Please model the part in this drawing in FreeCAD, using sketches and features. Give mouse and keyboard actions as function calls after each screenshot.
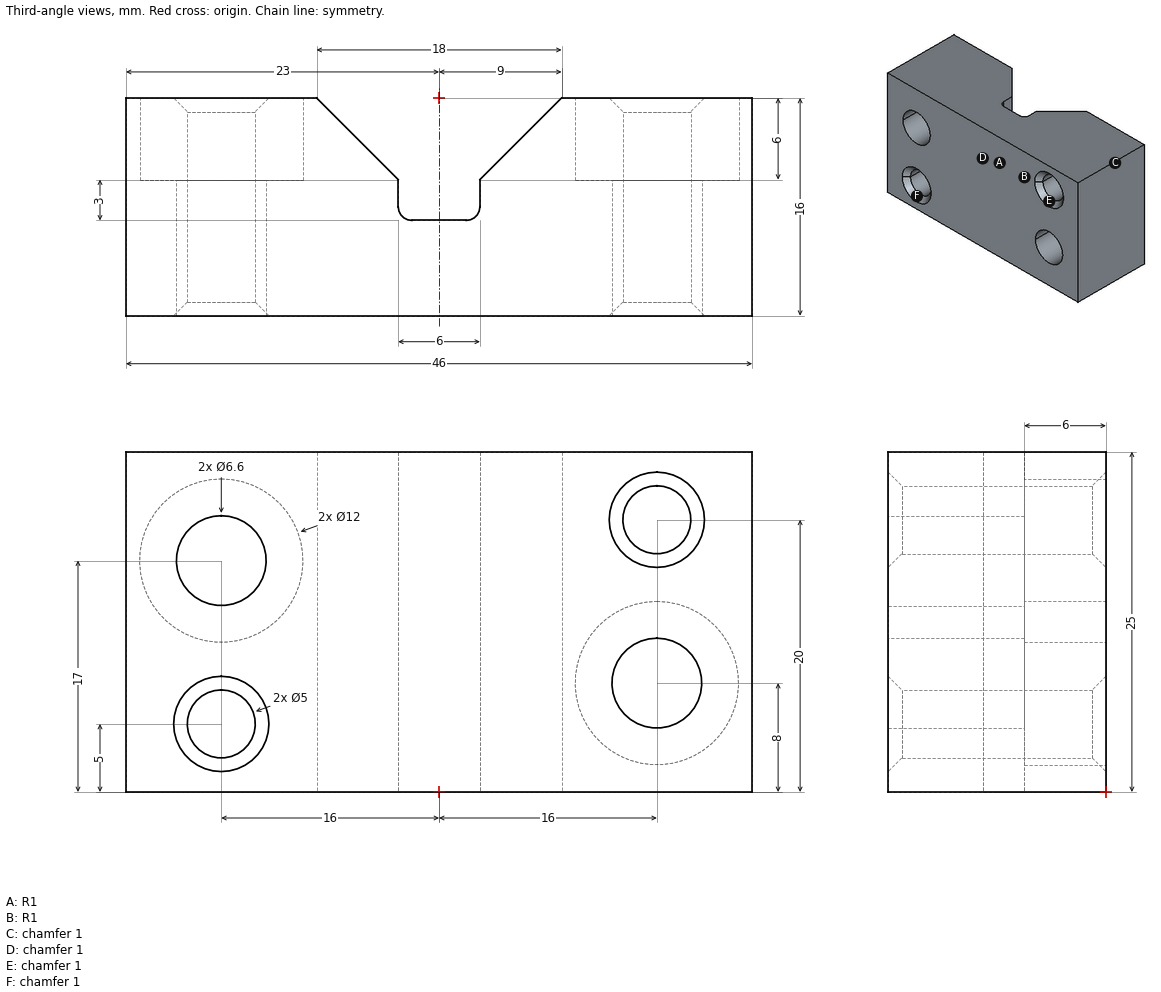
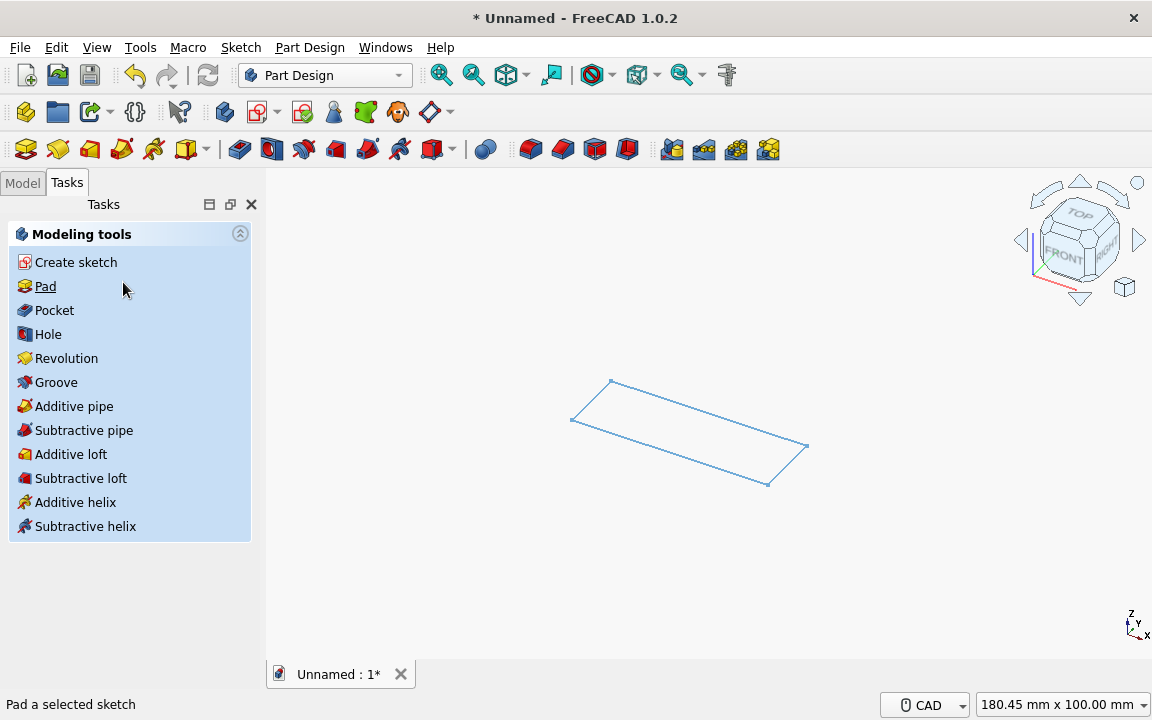
click(26, 150)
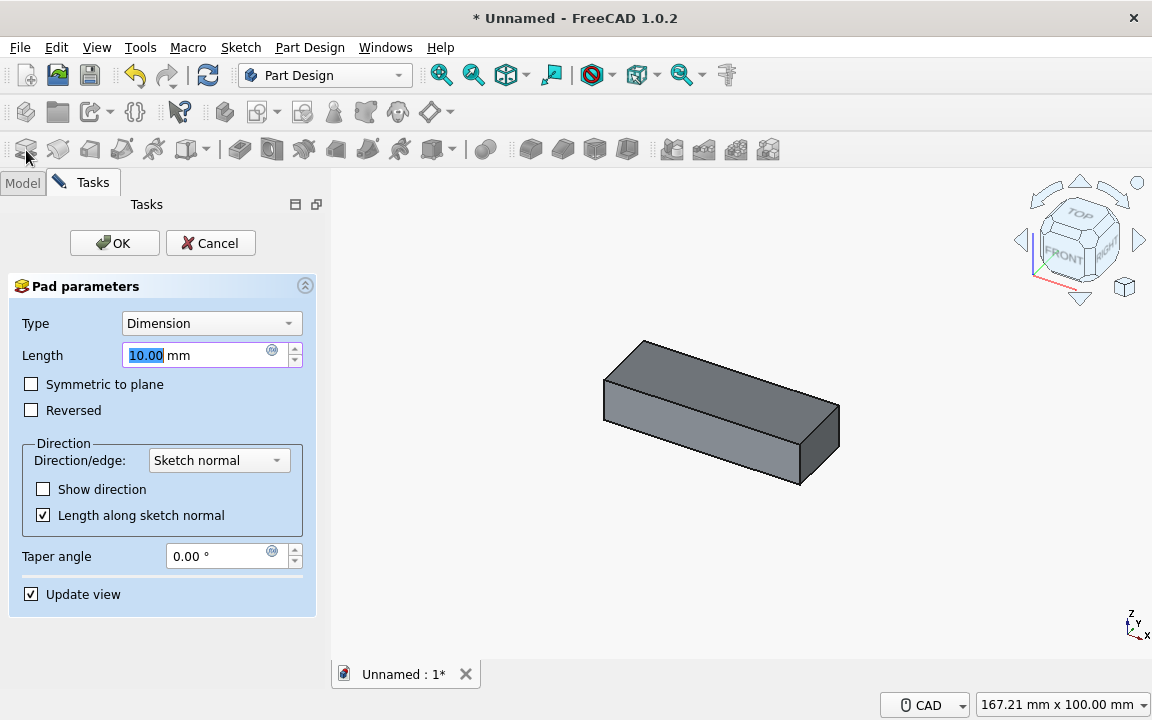
text(25)
key(Tab)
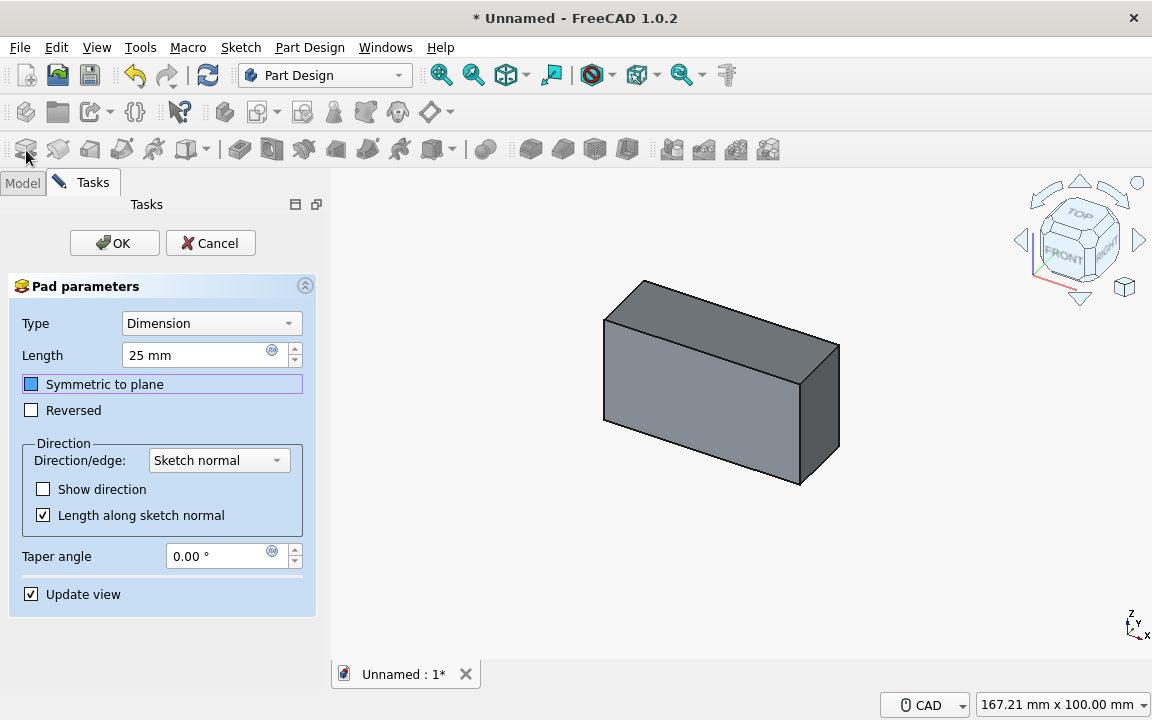
click(115, 243)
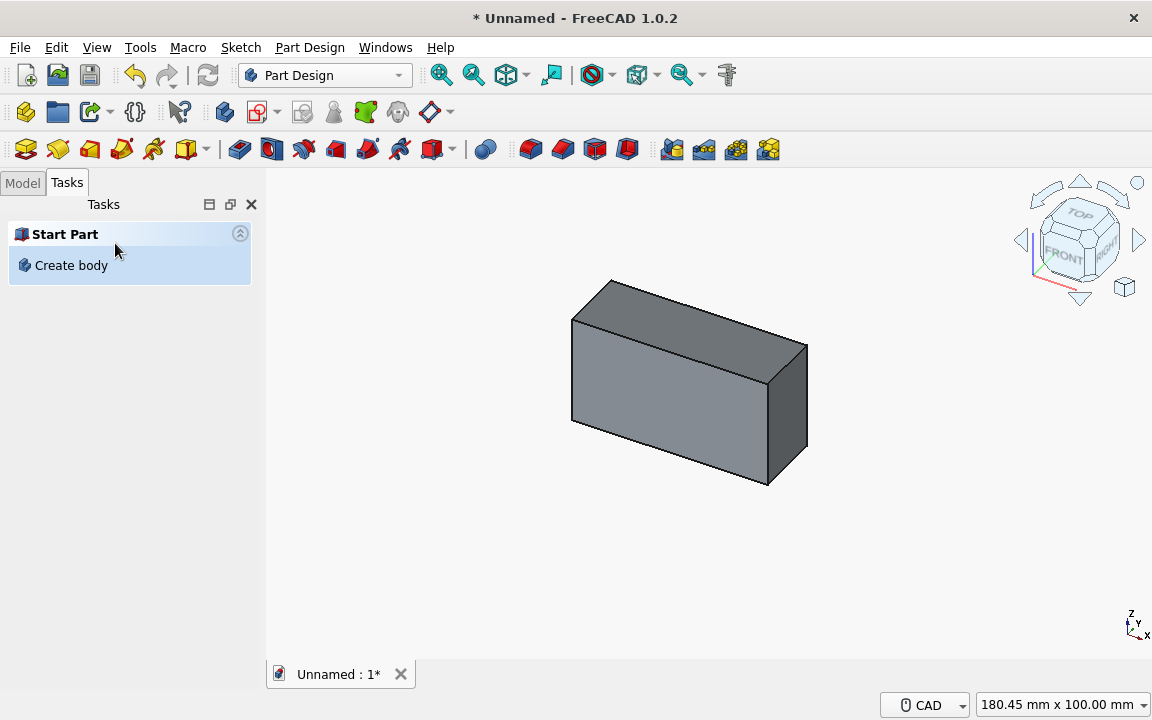
click(442, 76)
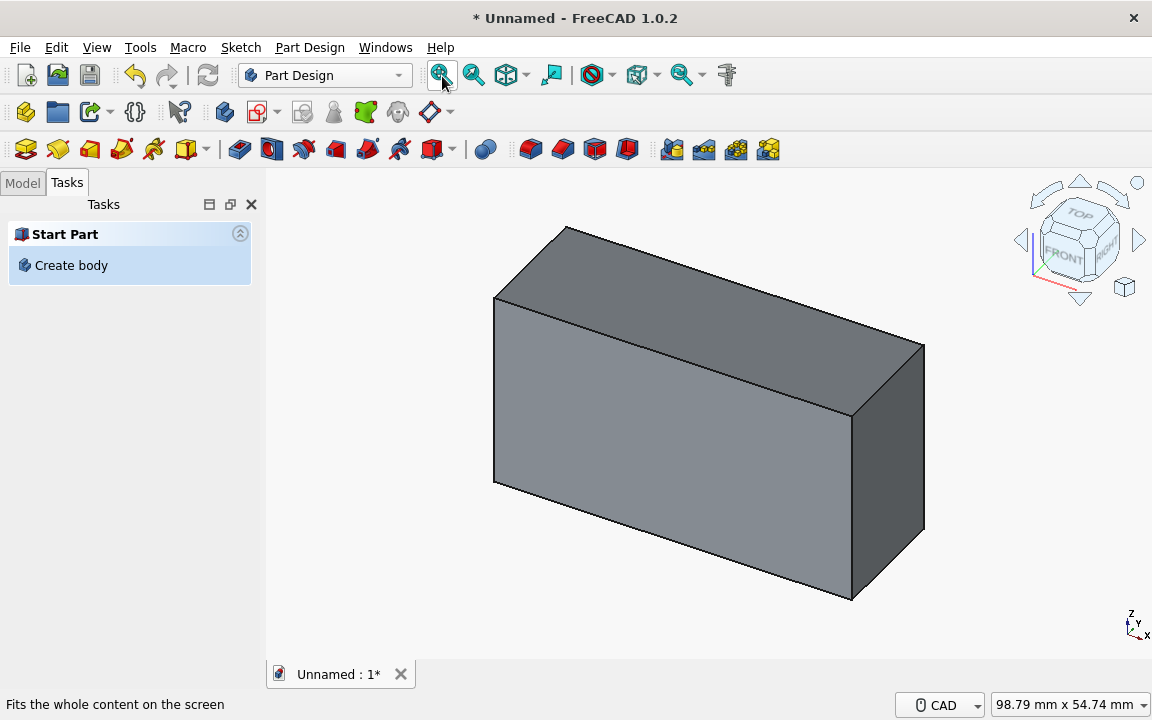
click(811, 354)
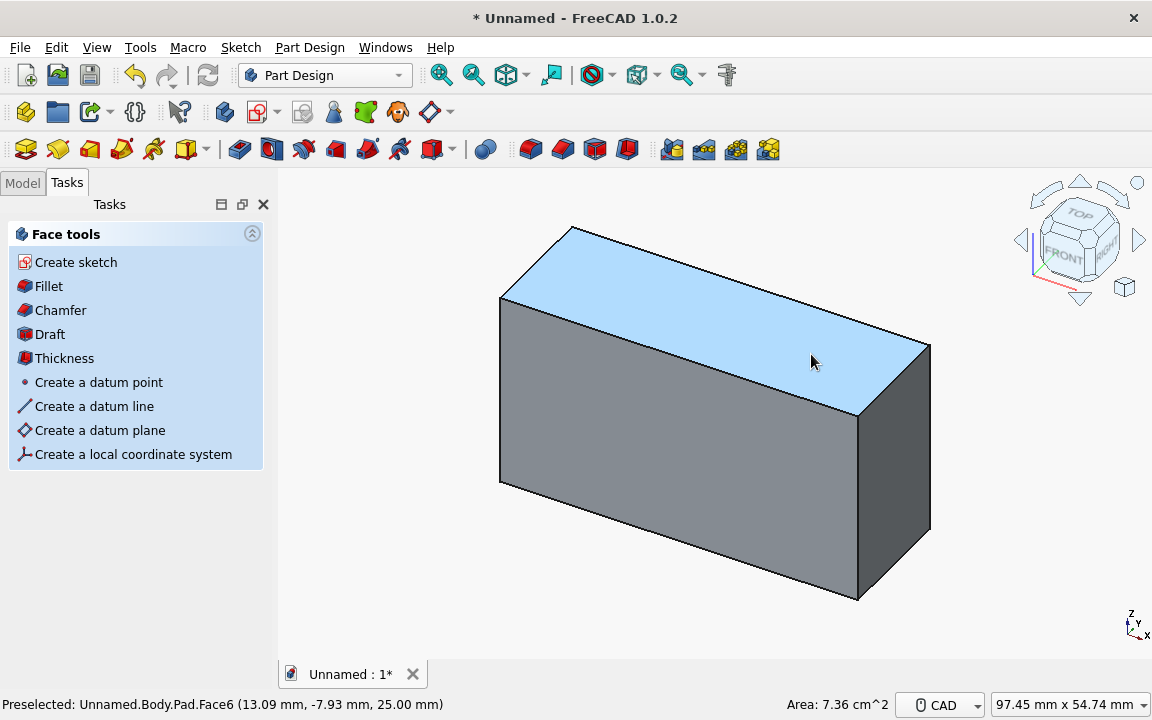
click(258, 112)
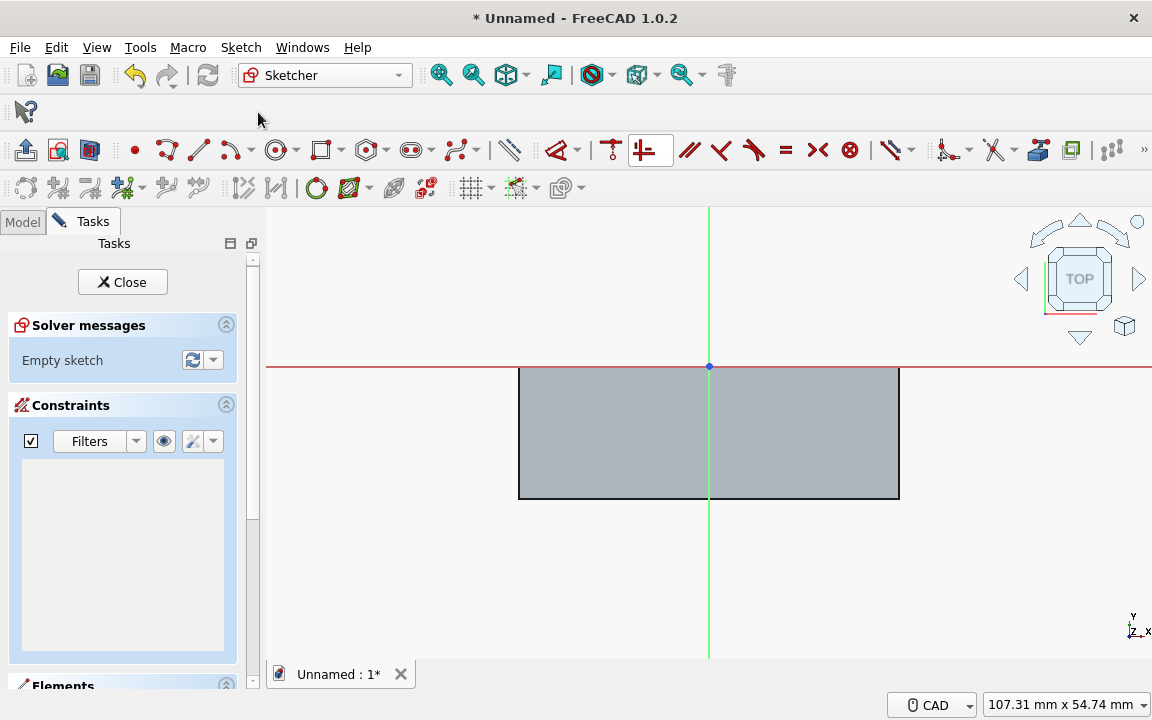
scroll(739, 392, up, 6)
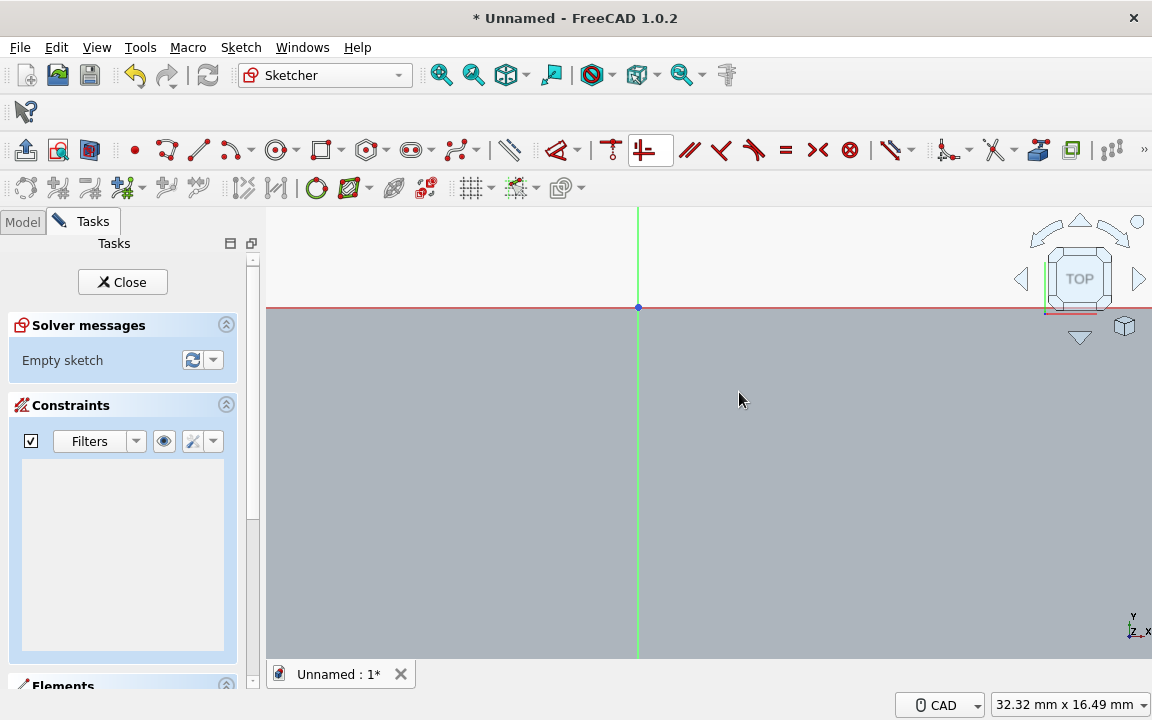
click(168, 150)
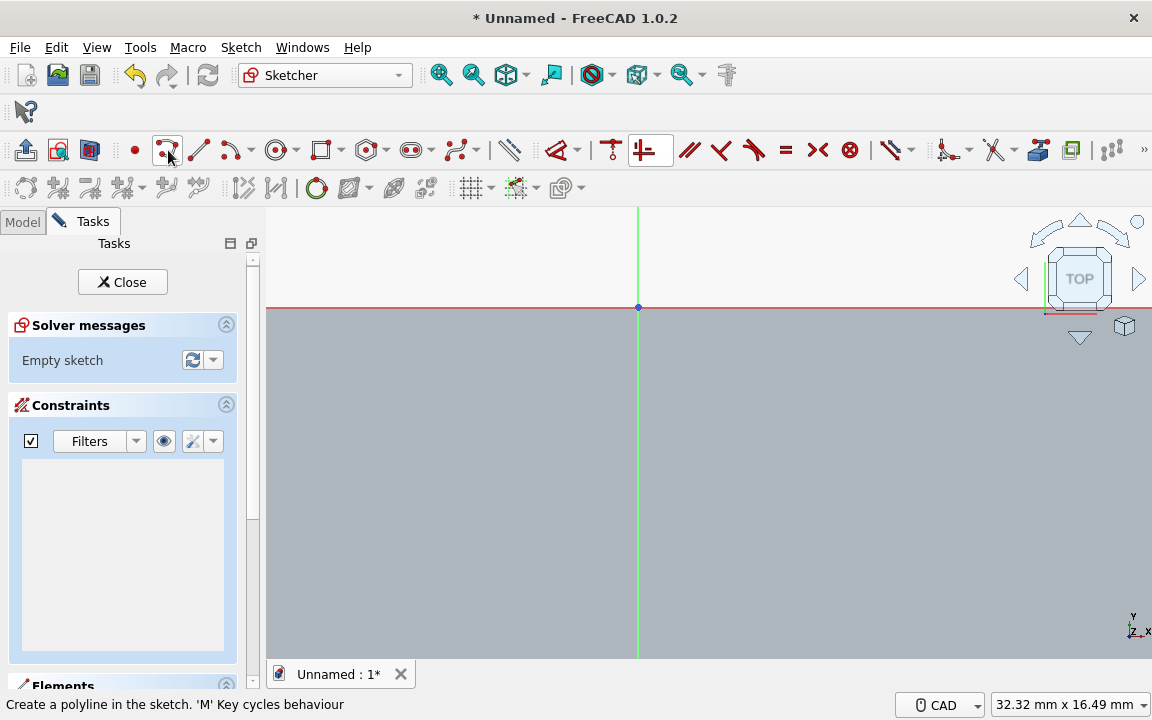
click(720, 472)
click(885, 308)
click(391, 317)
click(556, 472)
click(556, 555)
click(720, 555)
click(720, 473)
key(Escape)
key(Escape)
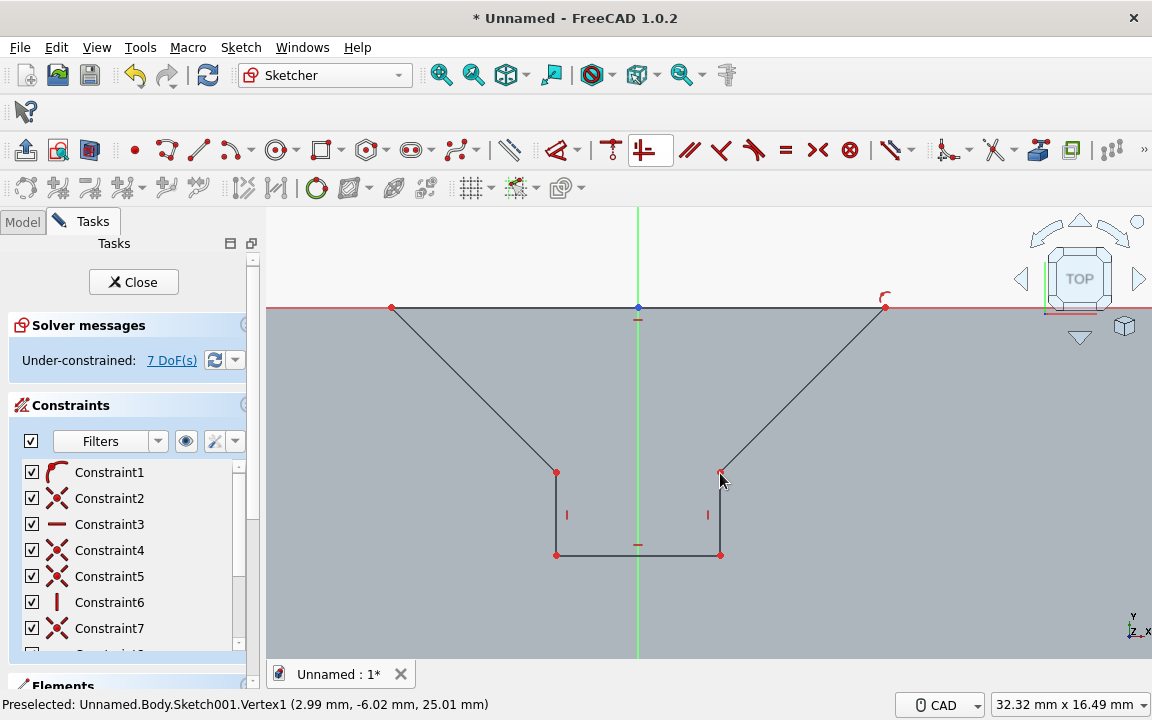
click(720, 473)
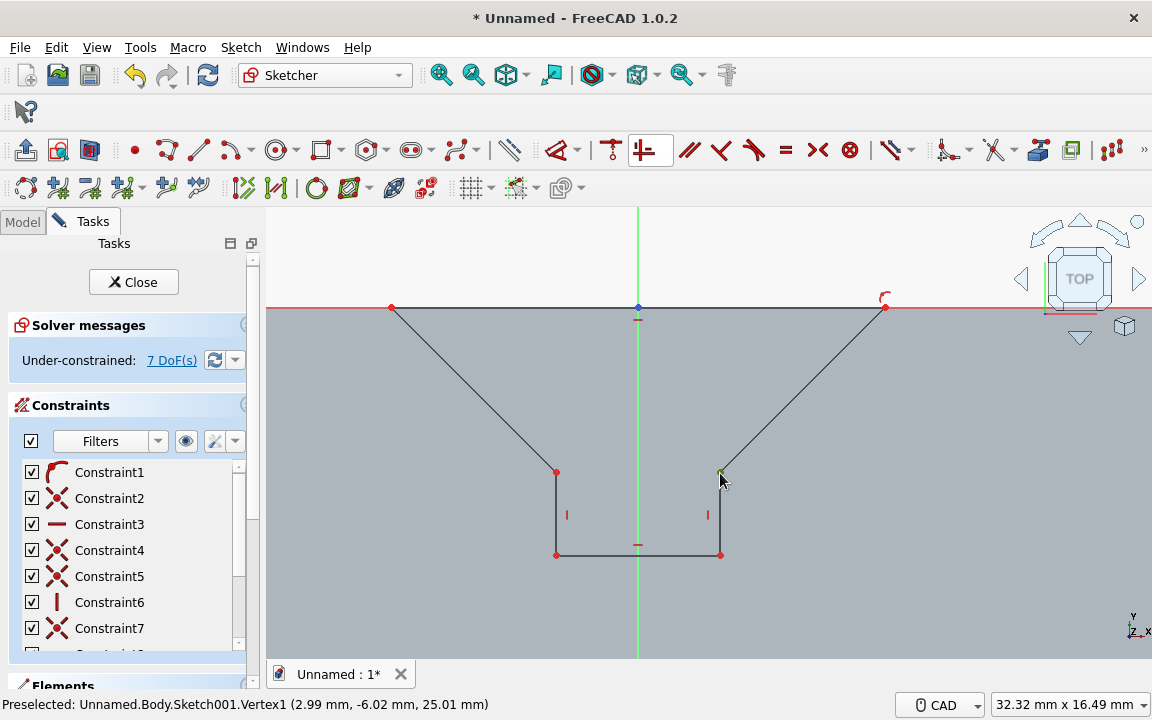
click(556, 473)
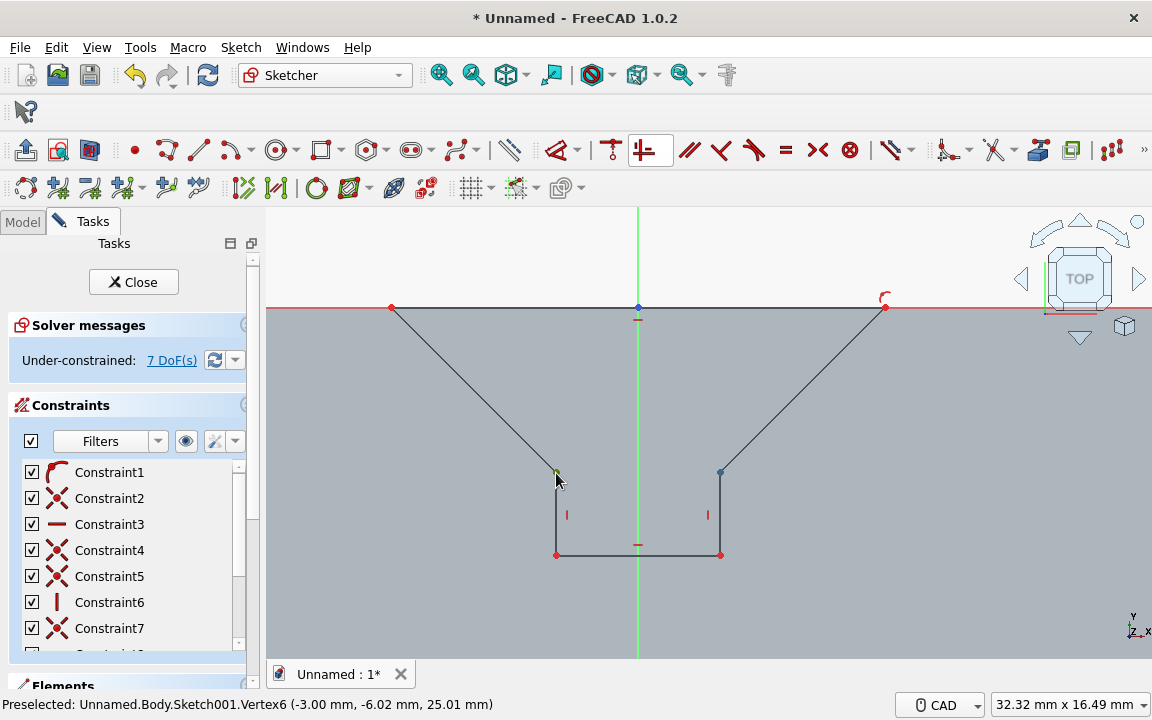
click(638, 603)